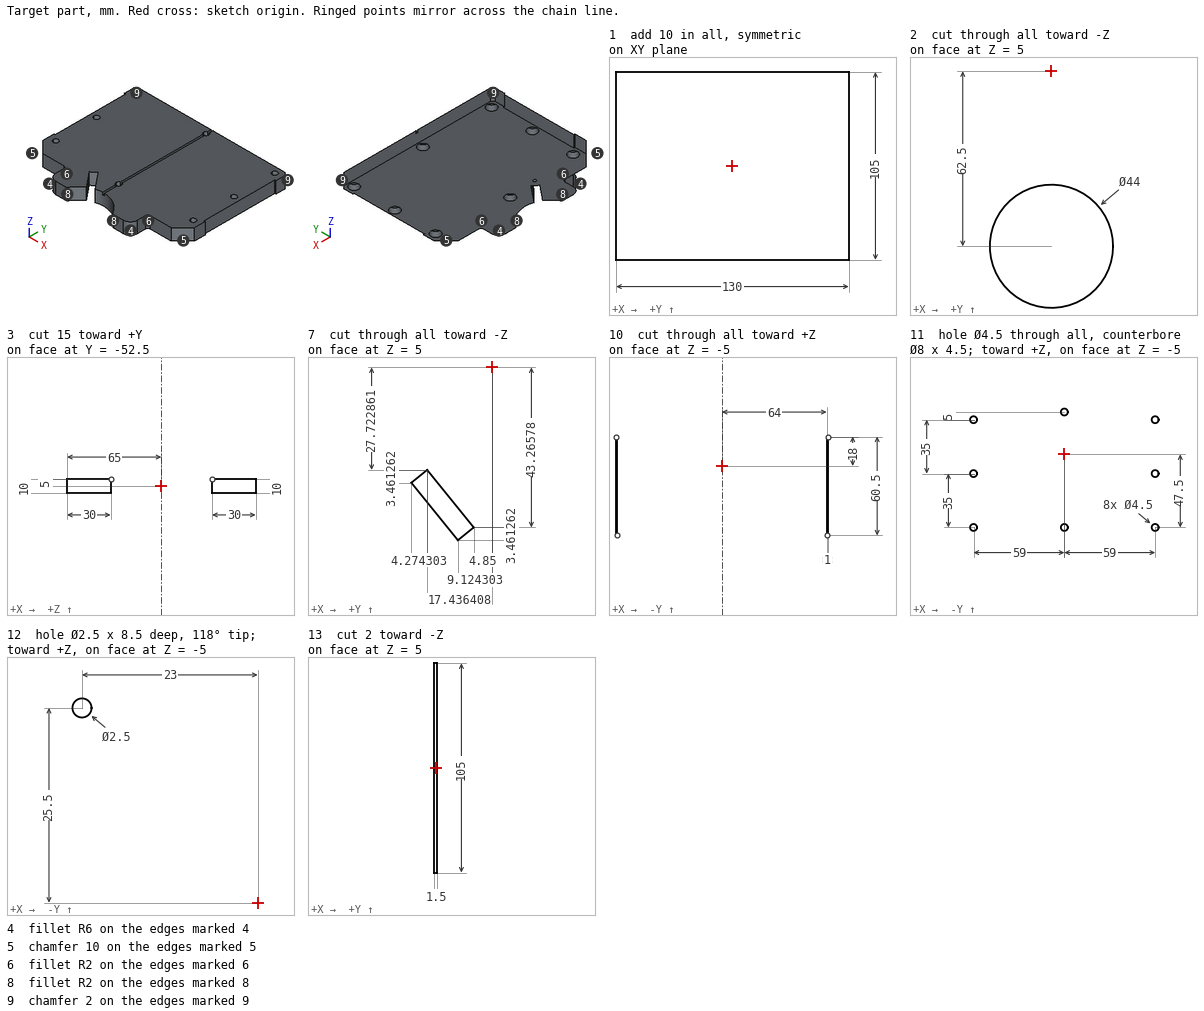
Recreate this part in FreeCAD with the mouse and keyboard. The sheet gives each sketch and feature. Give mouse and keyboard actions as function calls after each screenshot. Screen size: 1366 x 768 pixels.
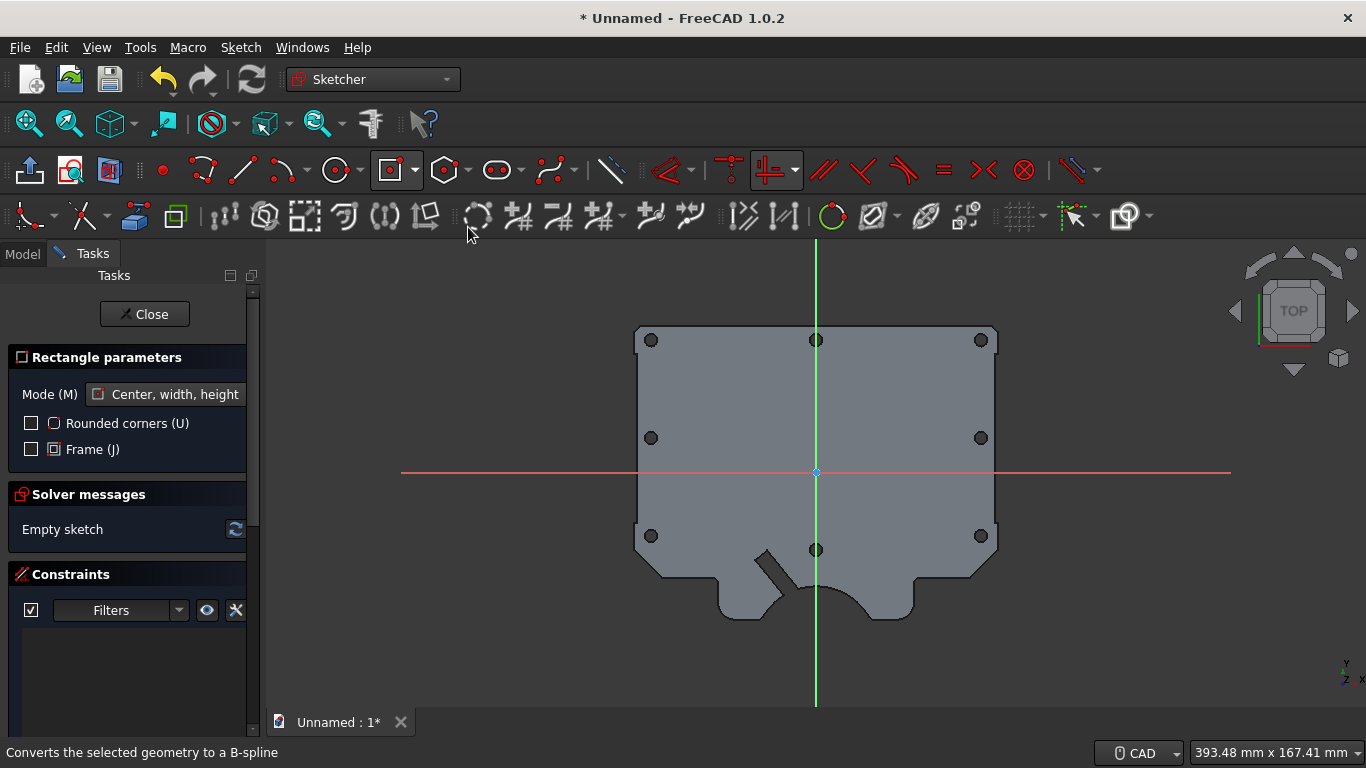
scroll(816, 473, up, 11)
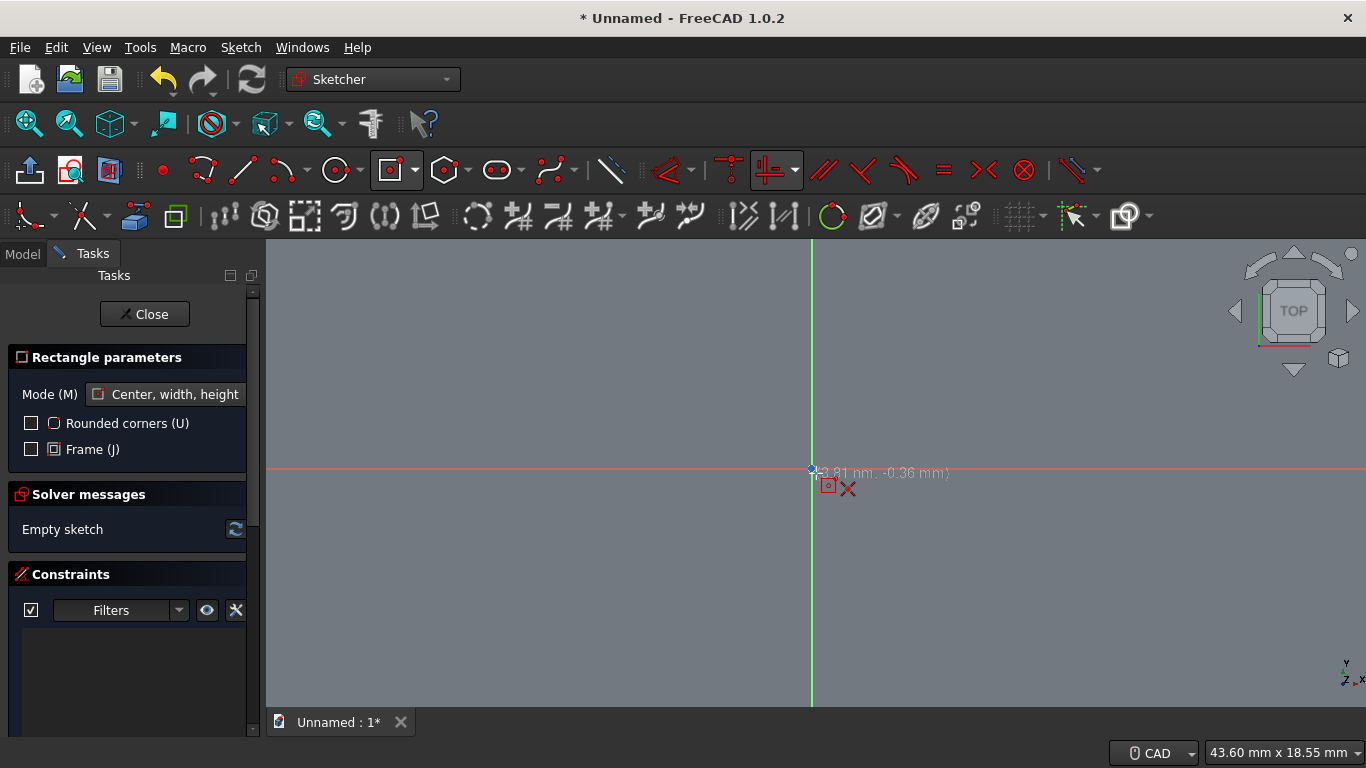
scroll(739, 474, down, 11)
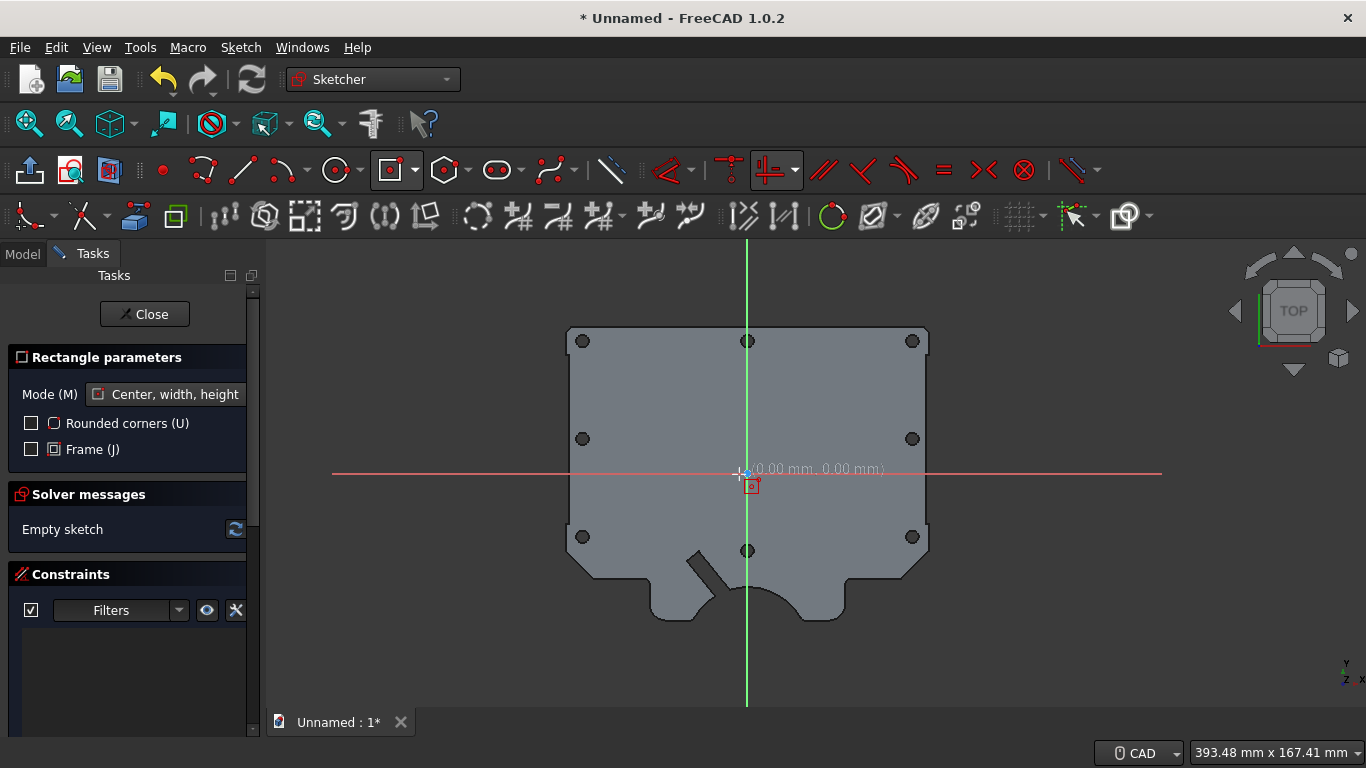
click(747, 474)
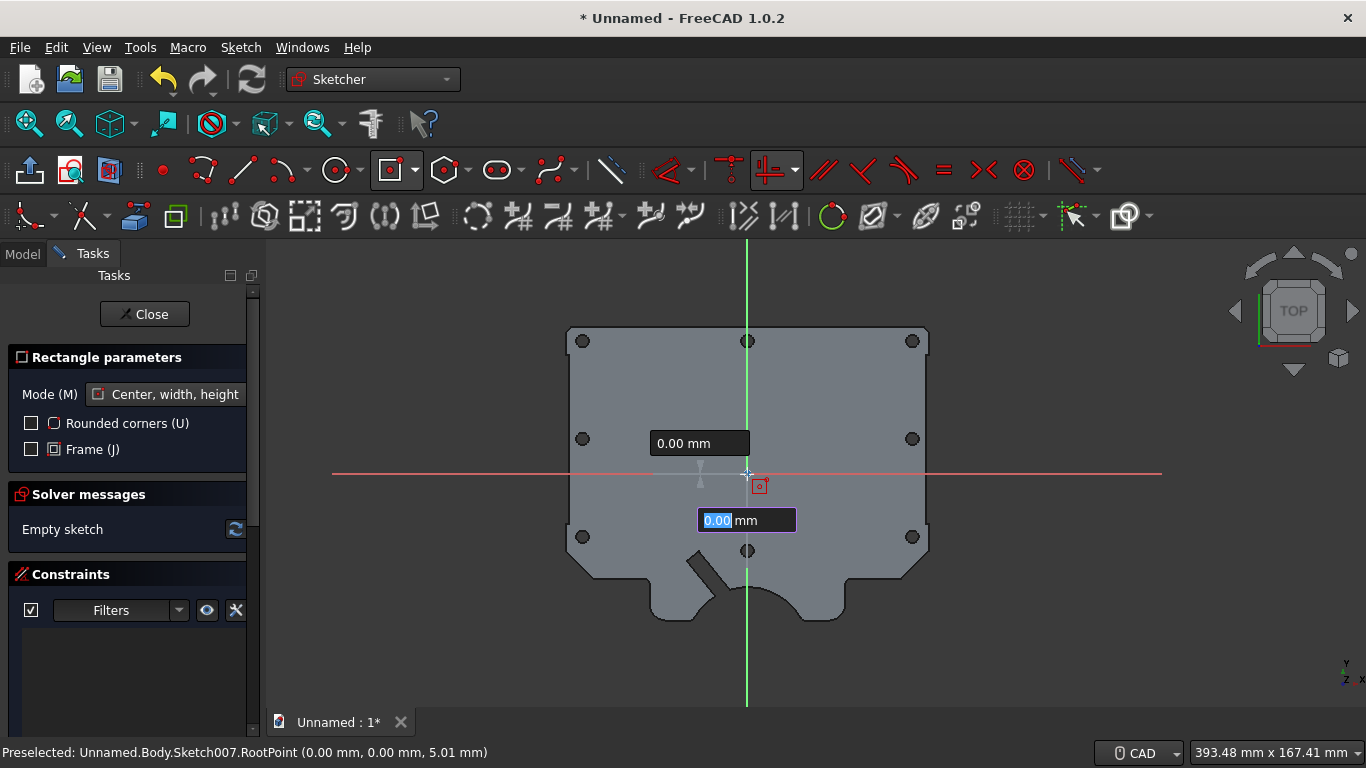
scroll(750, 327, up, 11)
move(743, 327)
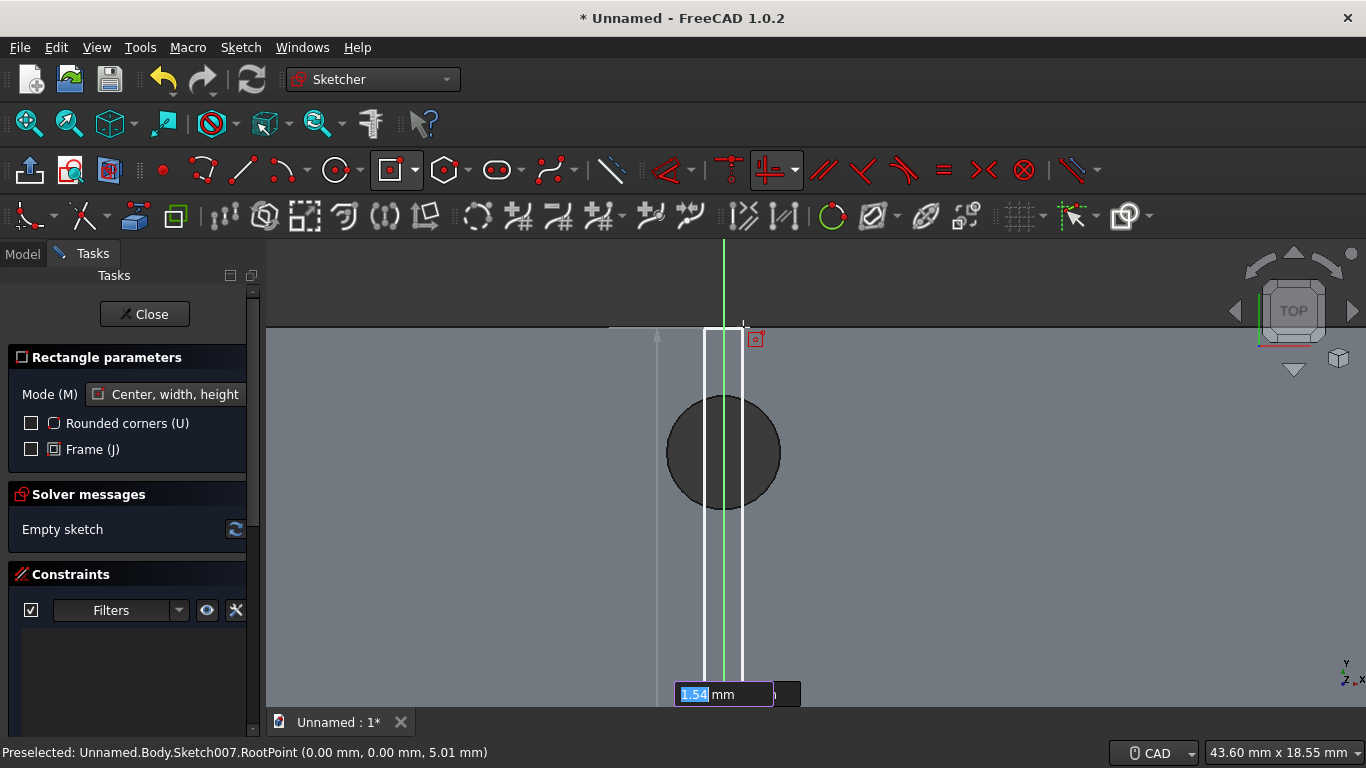
text(1.5)
key(Tab)
text(105)
key(Return)
key(Escape)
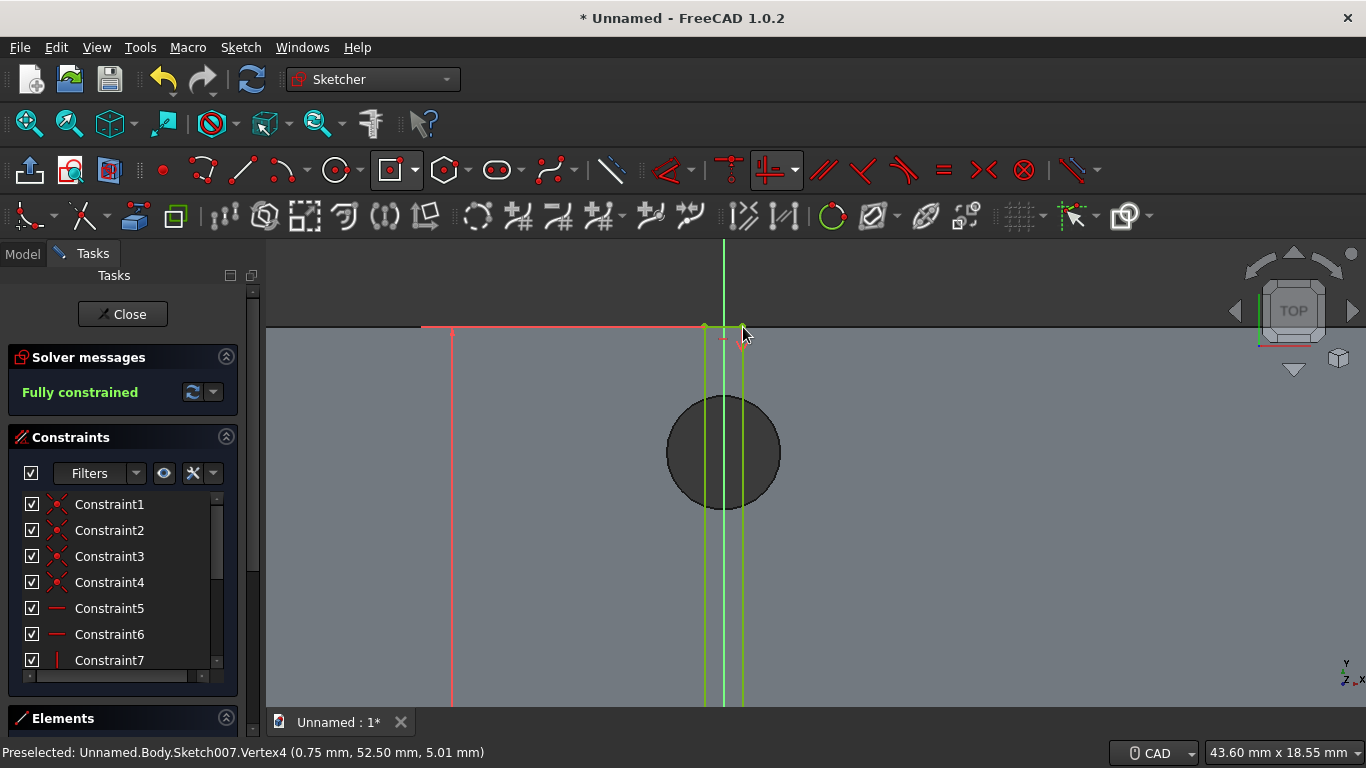
click(123, 314)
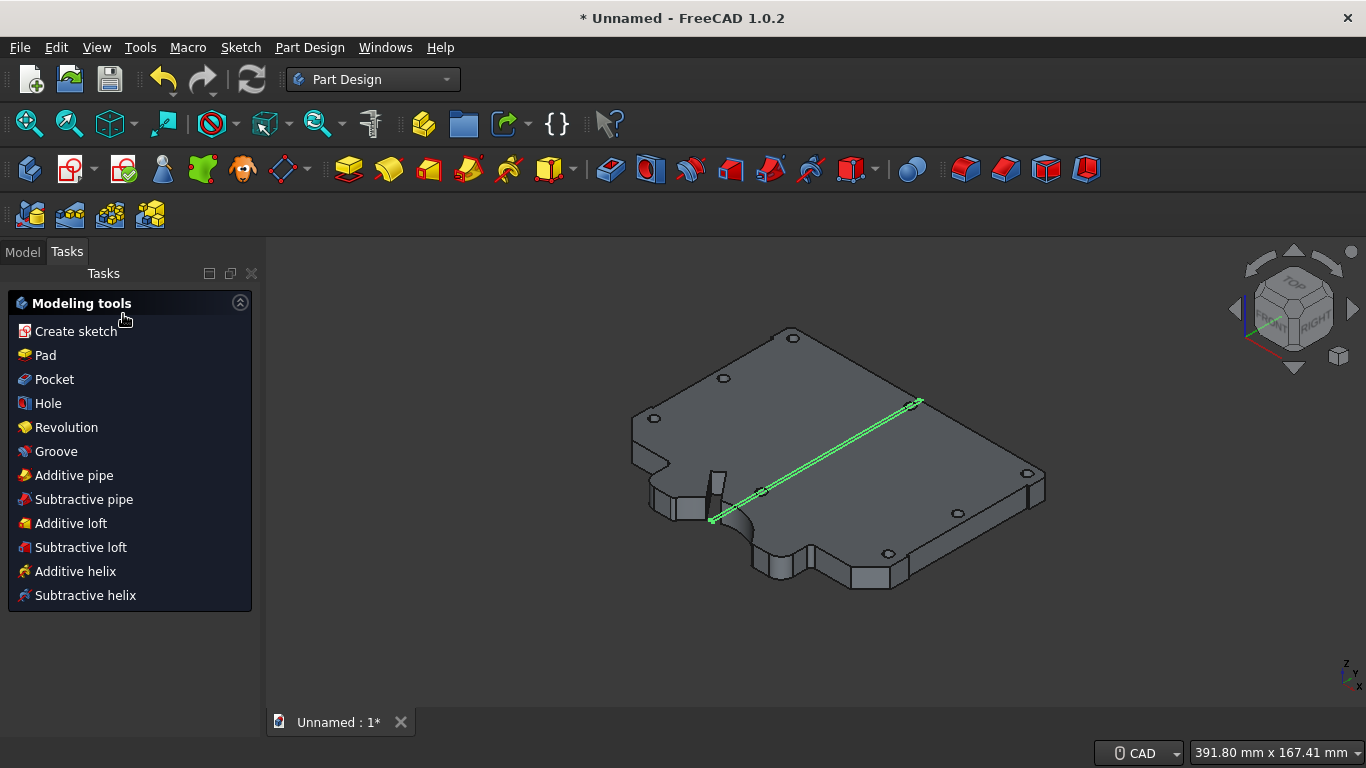
click(612, 170)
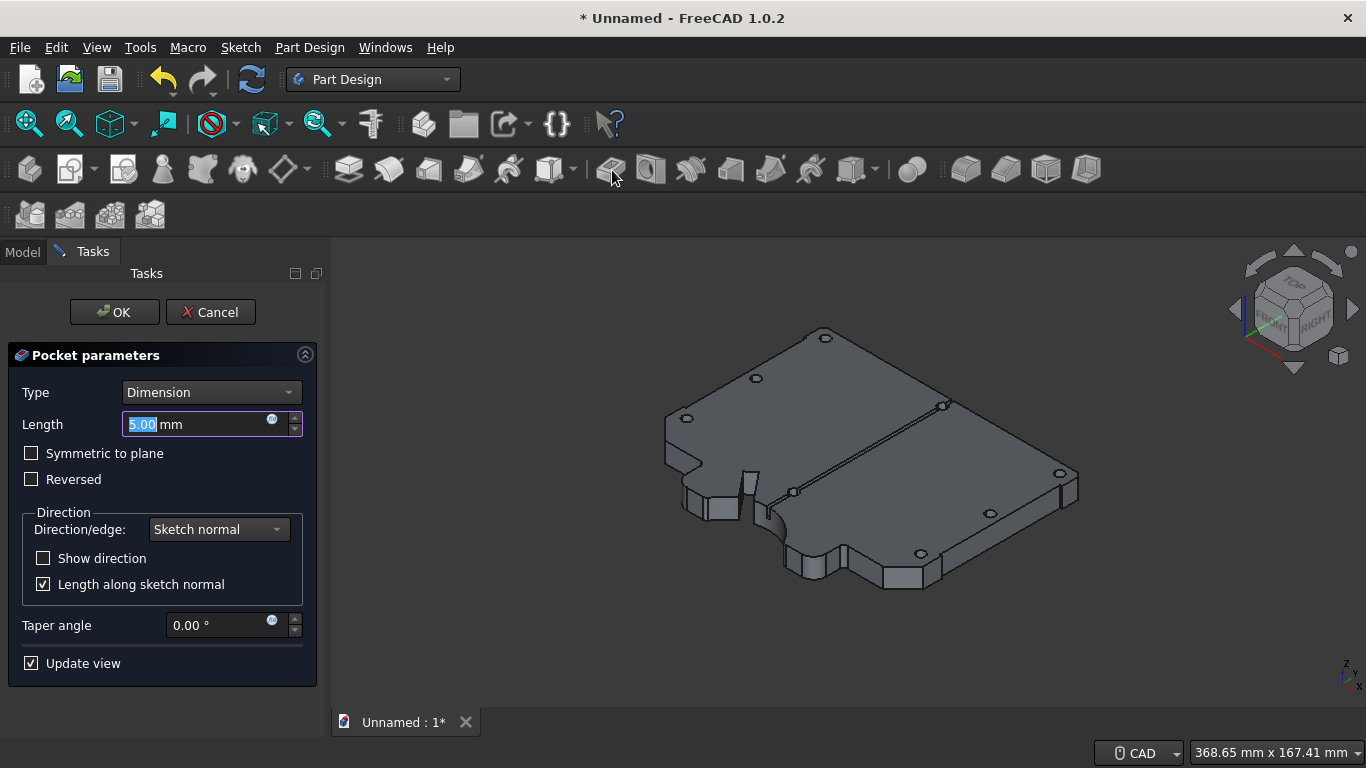
text(2)
key(Tab)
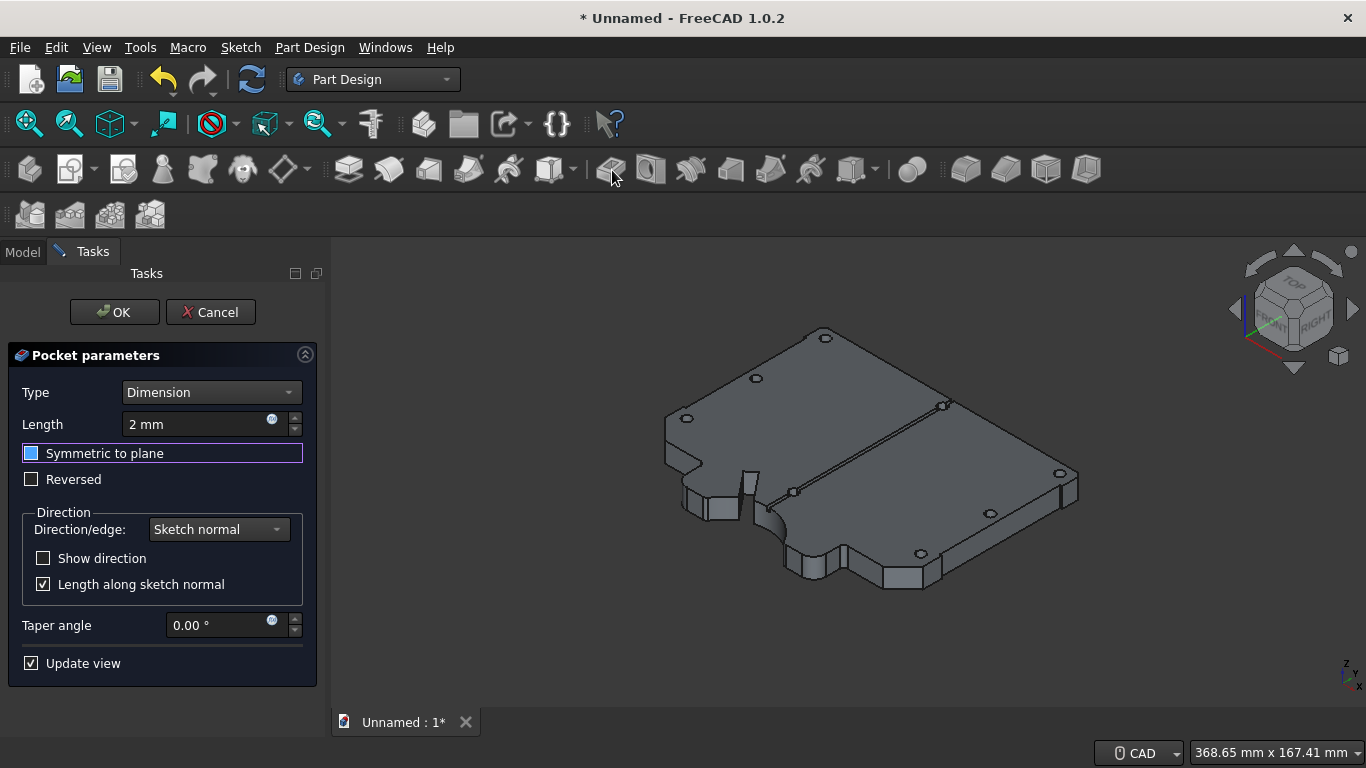
click(115, 312)